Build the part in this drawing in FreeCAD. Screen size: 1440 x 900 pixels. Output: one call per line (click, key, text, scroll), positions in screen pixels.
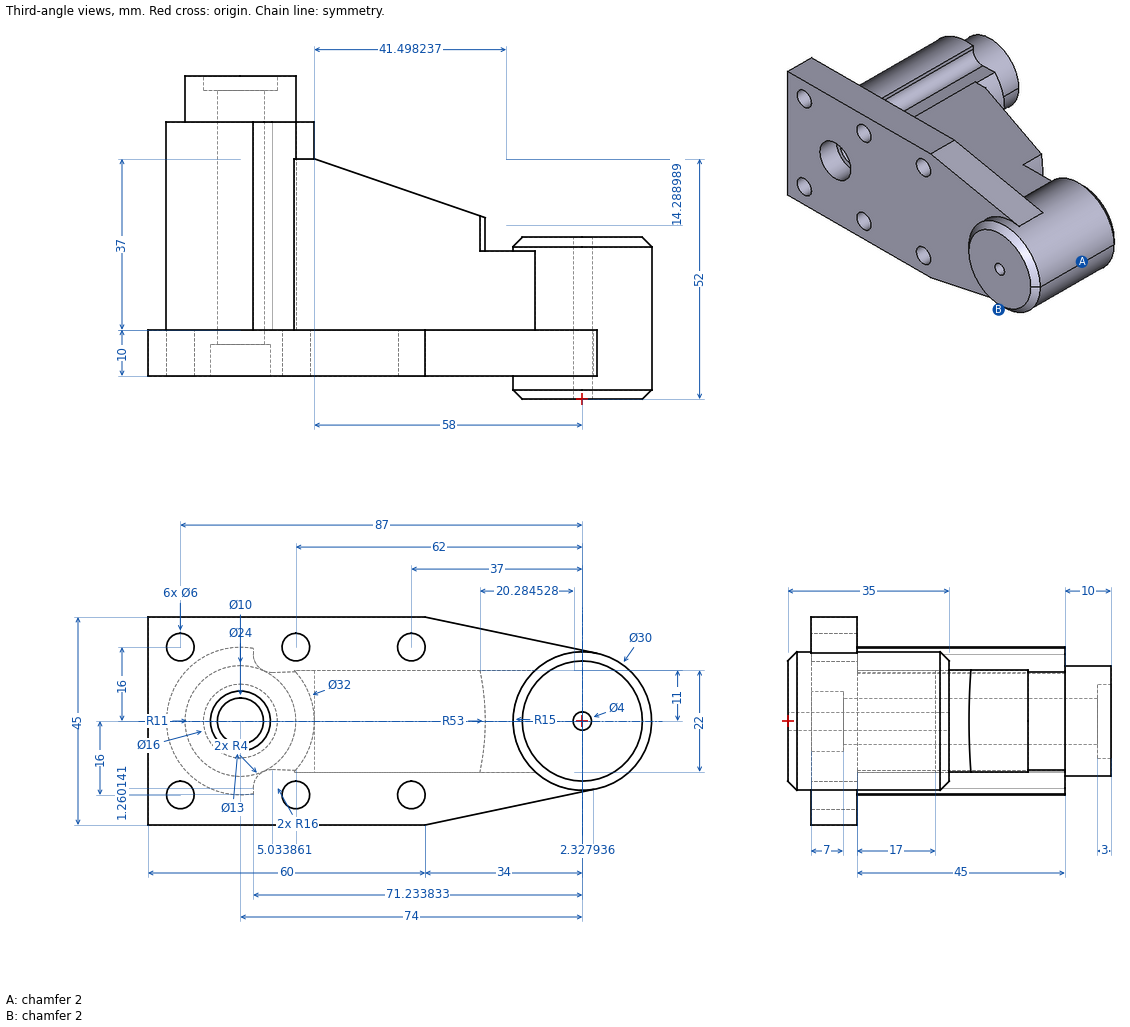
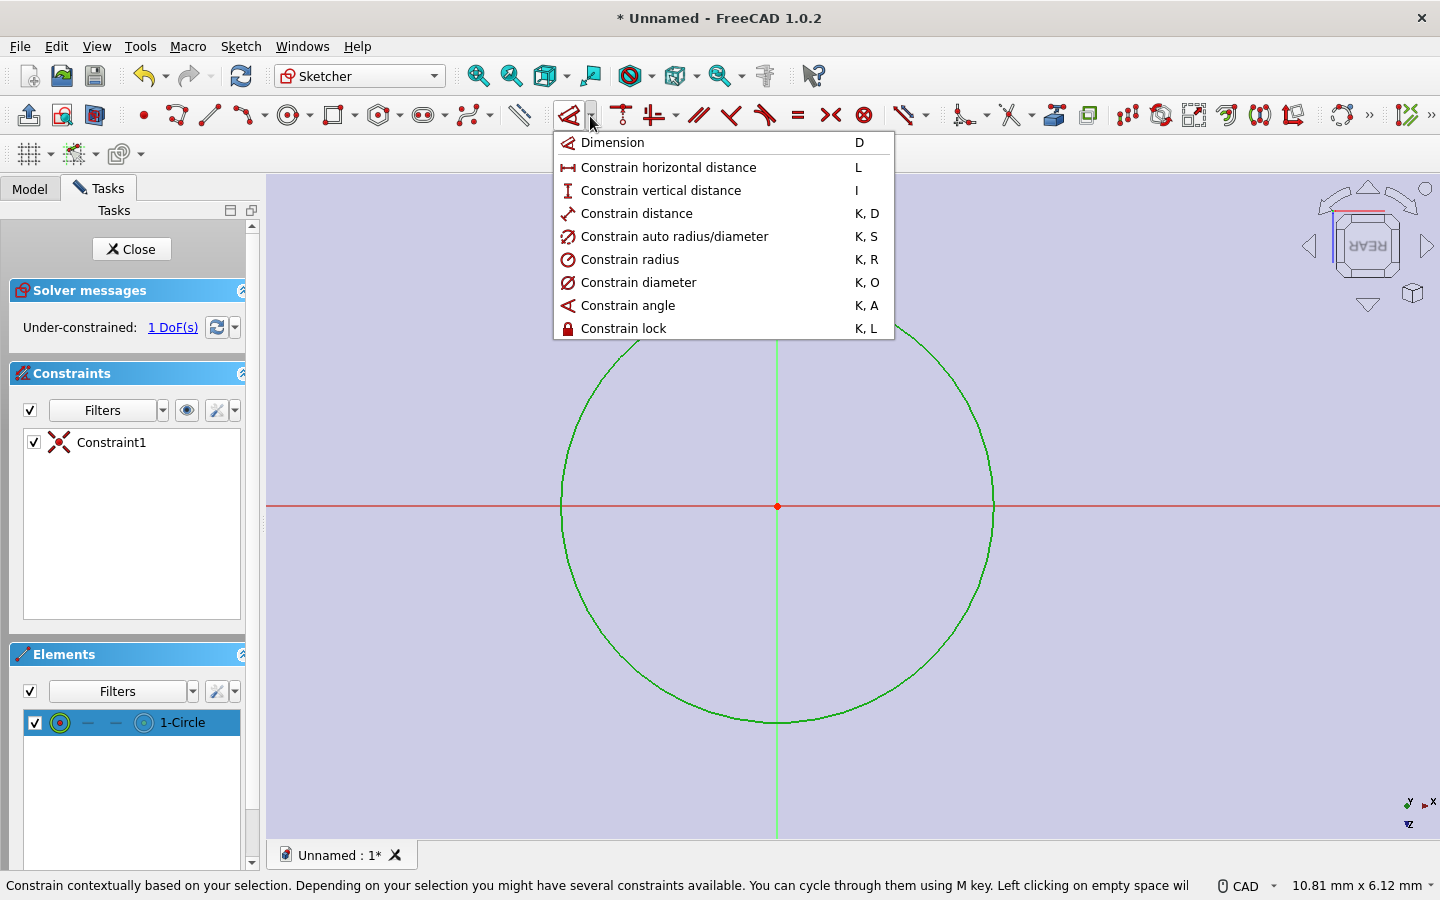
click(724, 282)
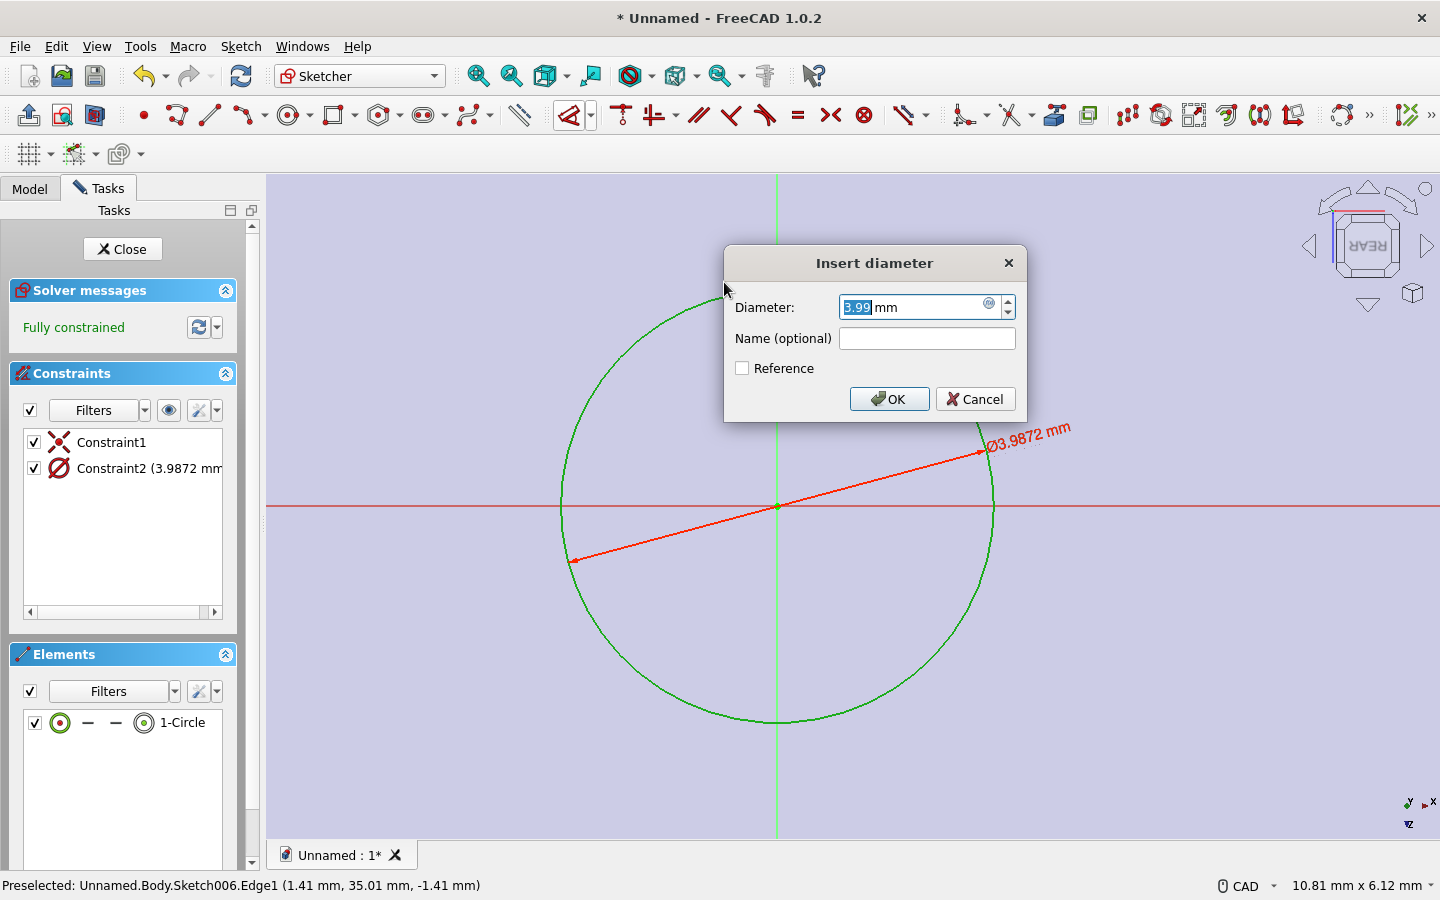
text(4)
key(Return)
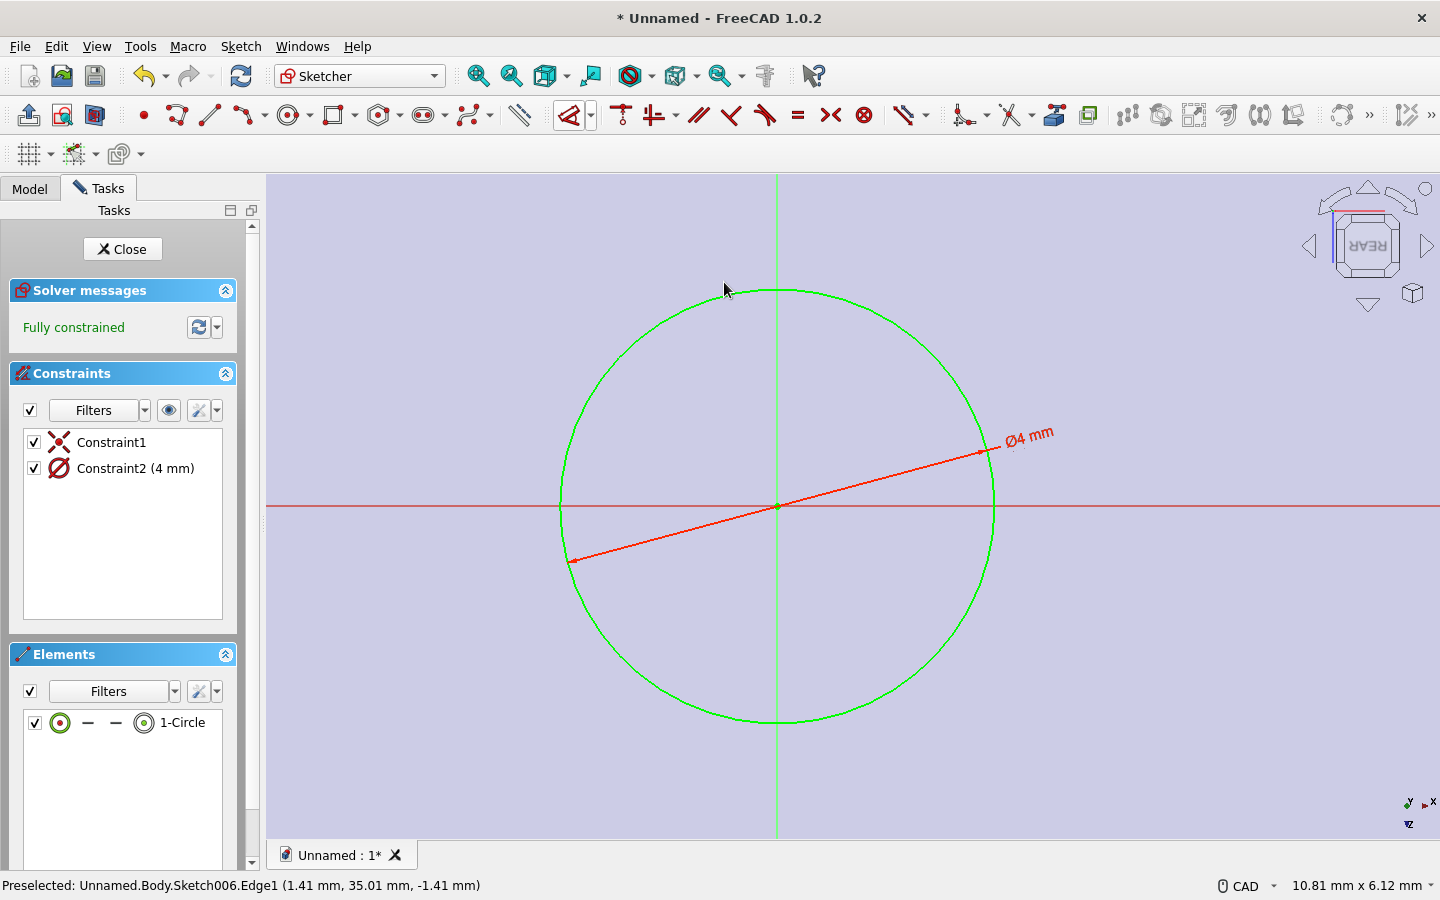
click(123, 249)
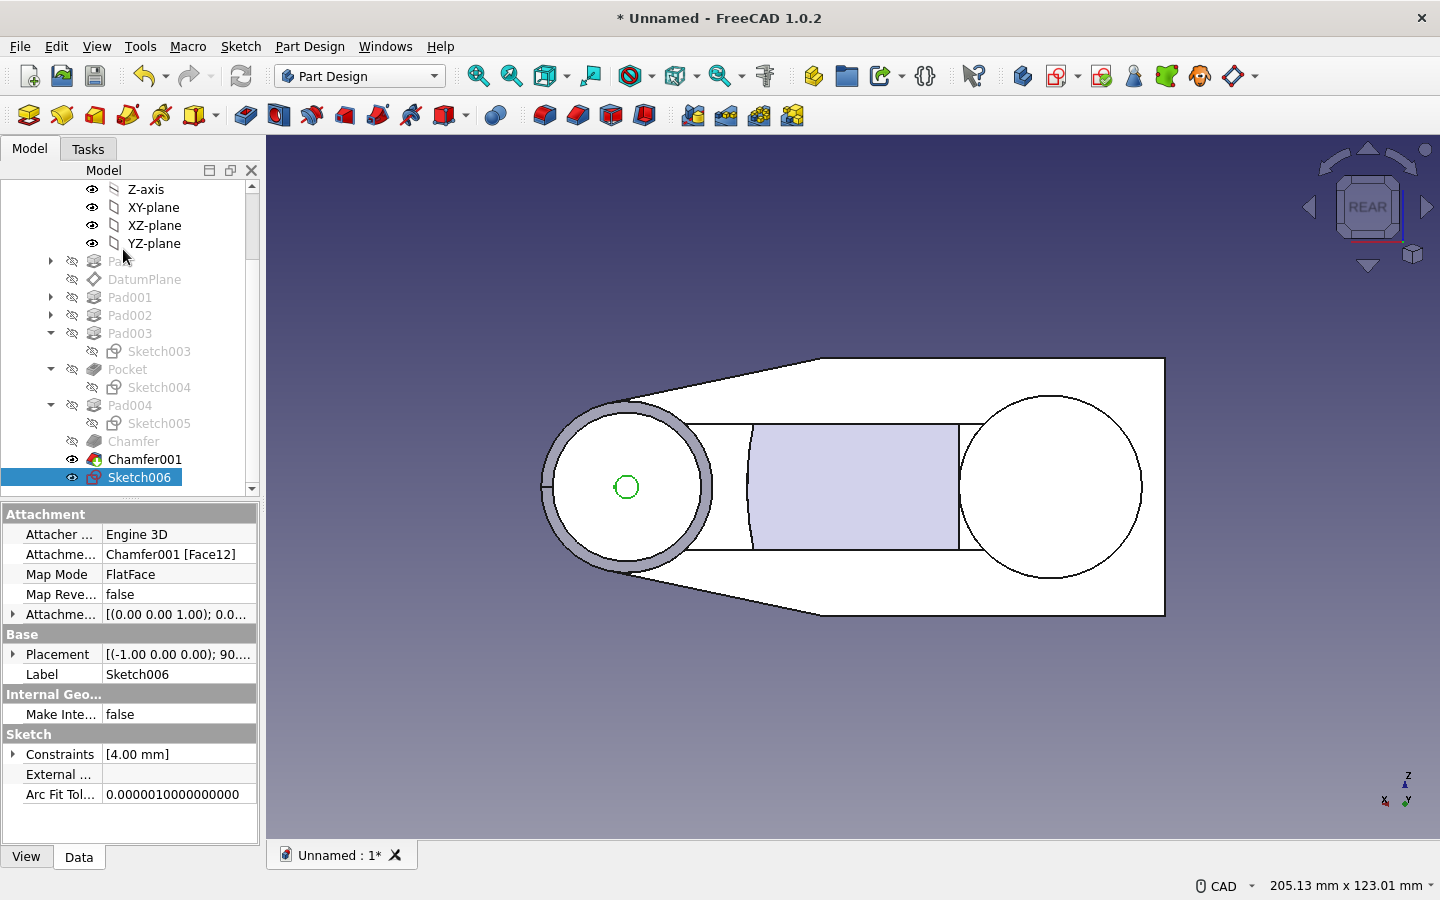
click(246, 116)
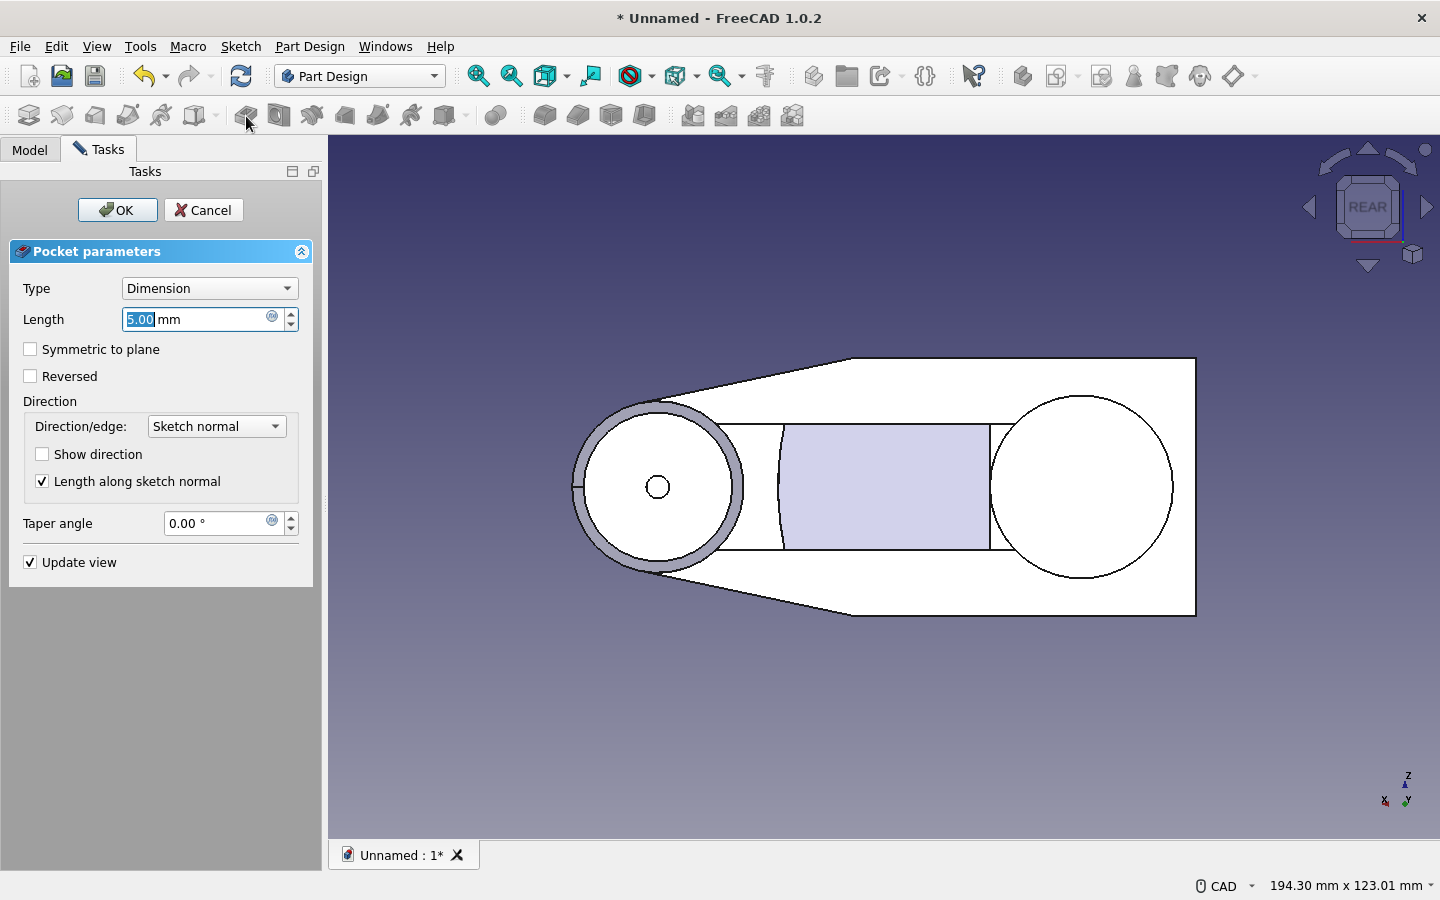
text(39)
key(Tab)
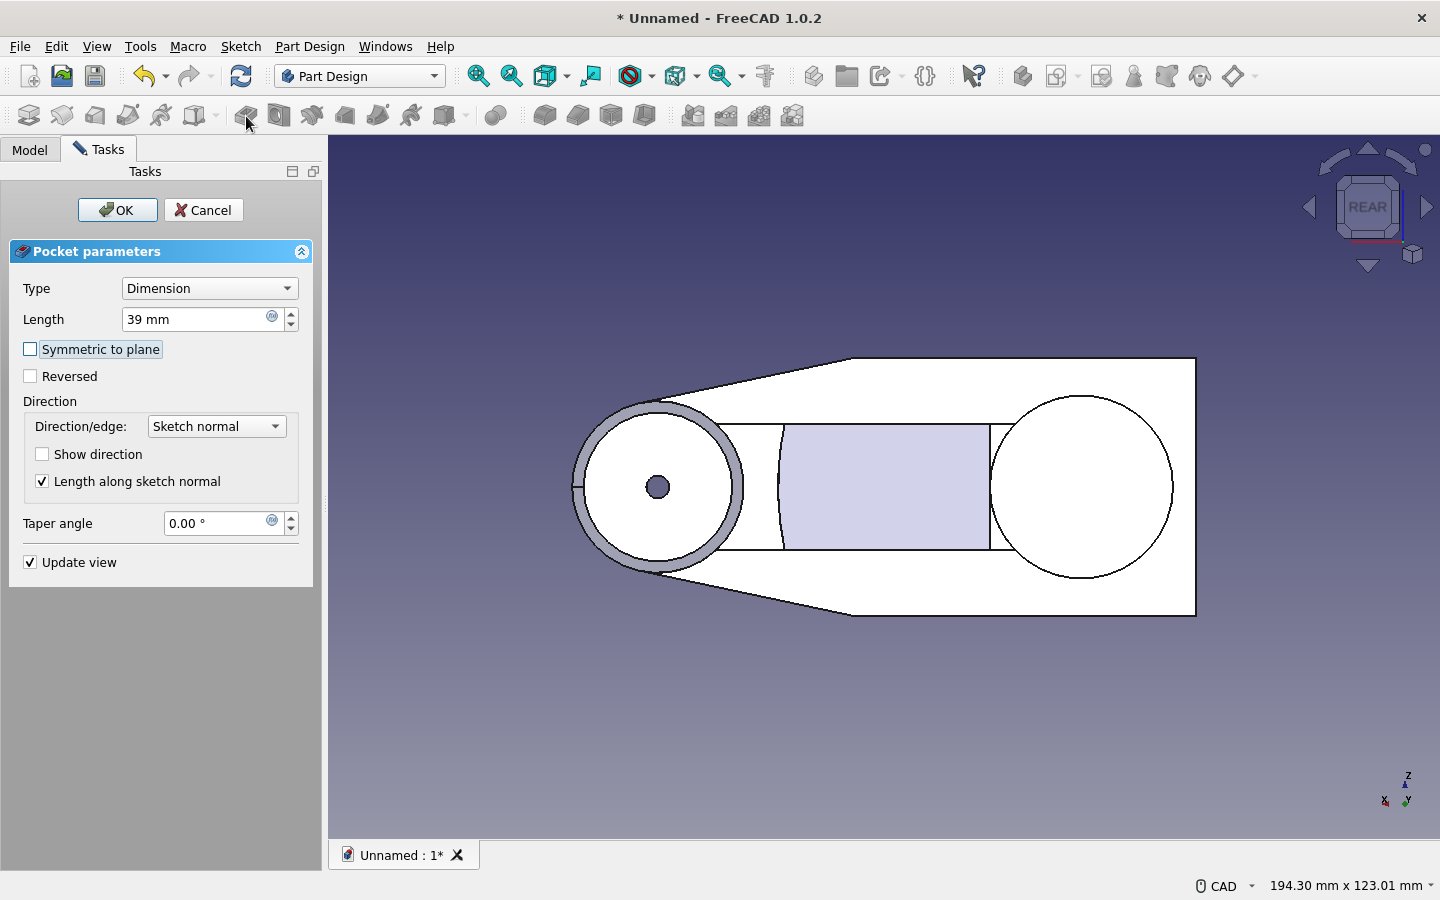
click(118, 210)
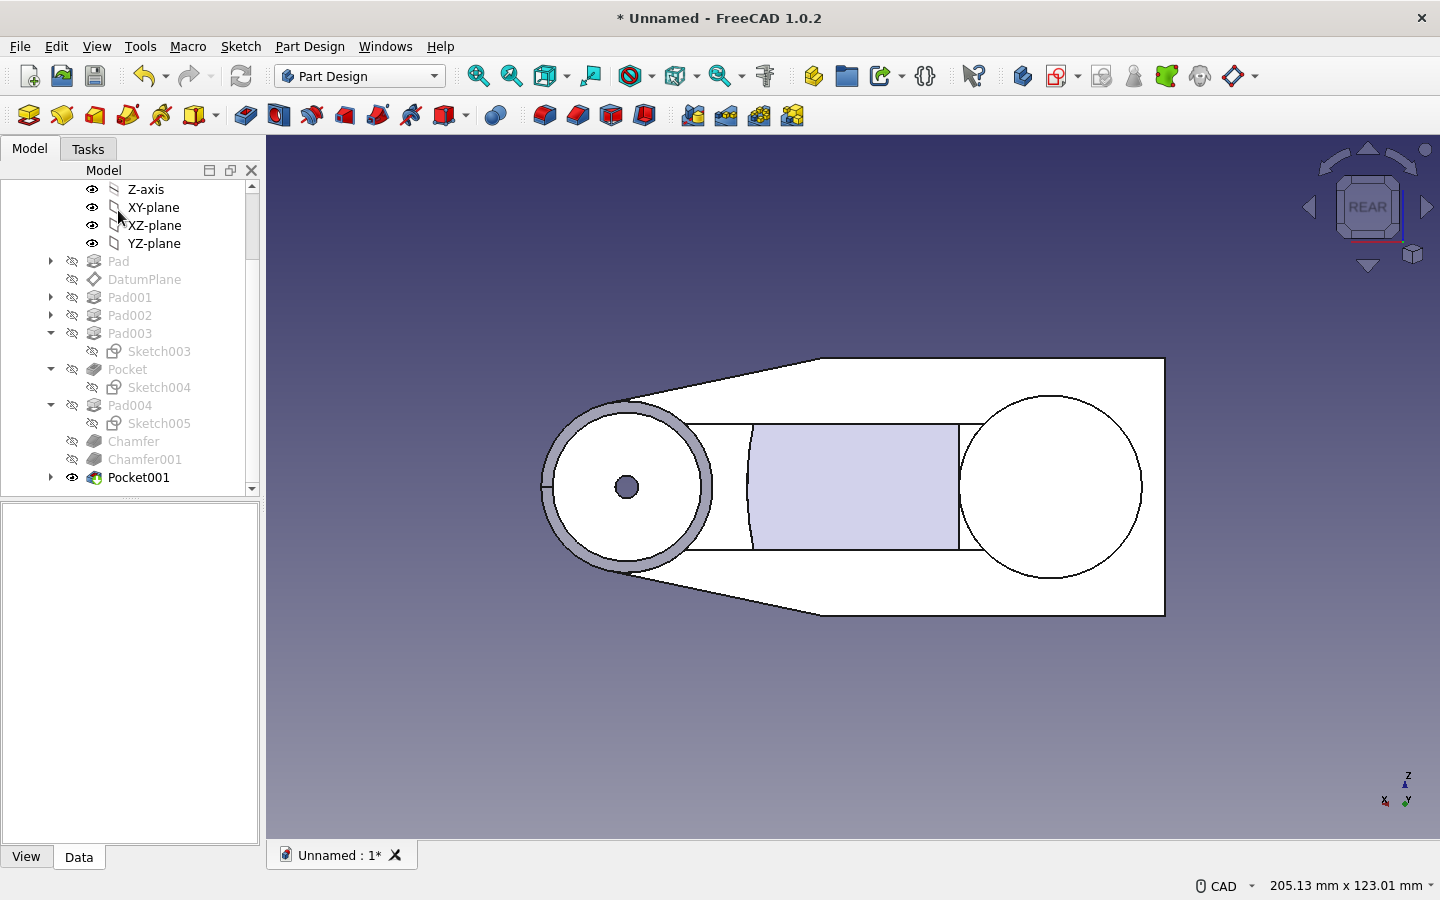
click(1050, 486)